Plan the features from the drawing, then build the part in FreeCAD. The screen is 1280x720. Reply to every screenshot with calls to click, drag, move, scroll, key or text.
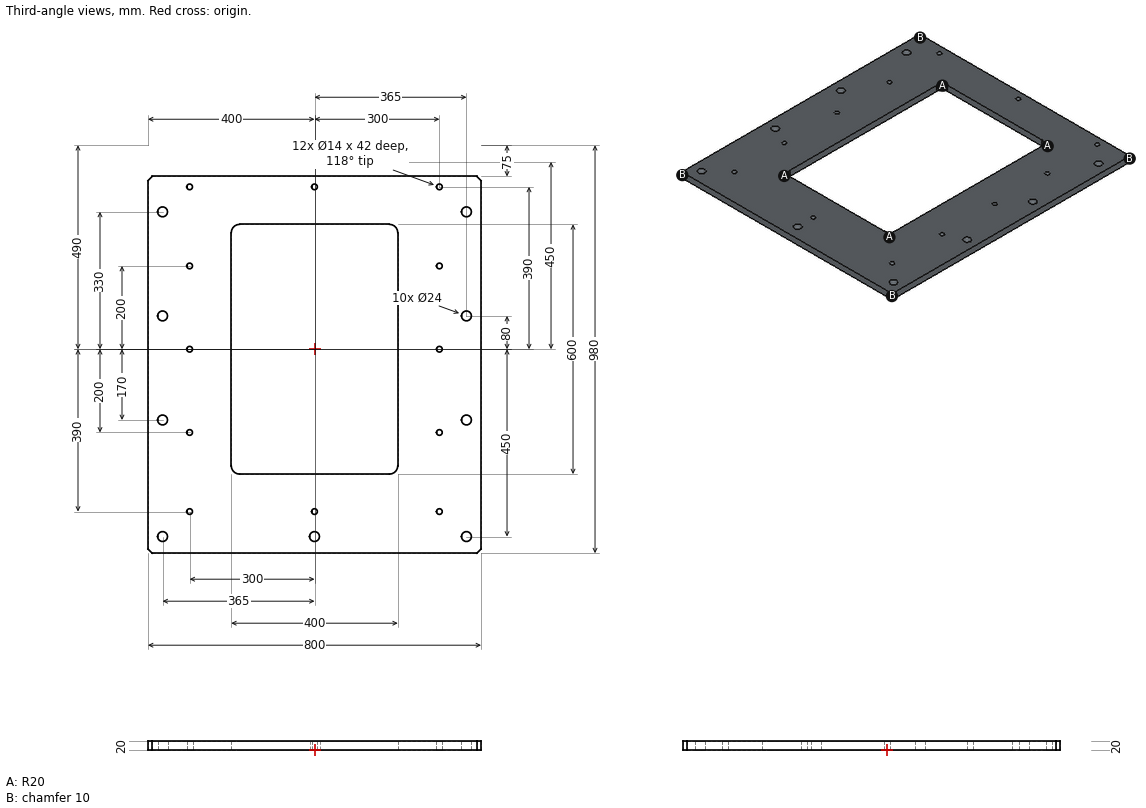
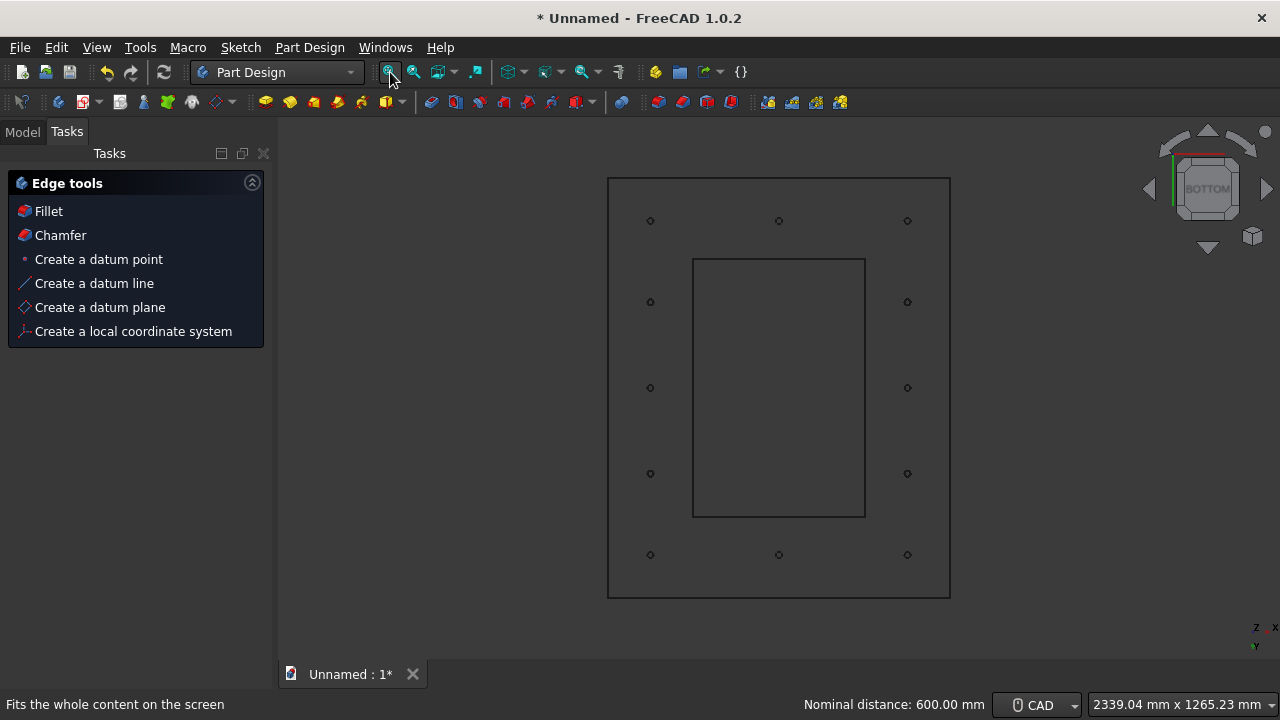
scroll(693, 258, up, 8)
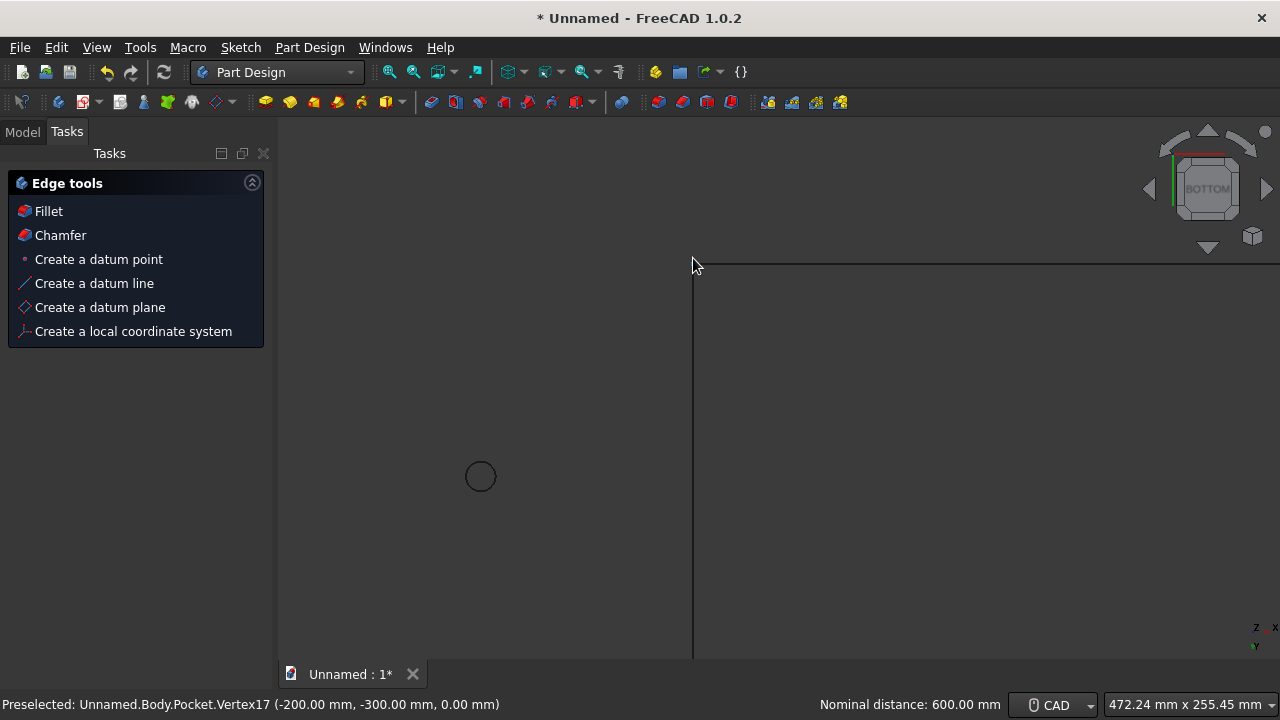
click(390, 72)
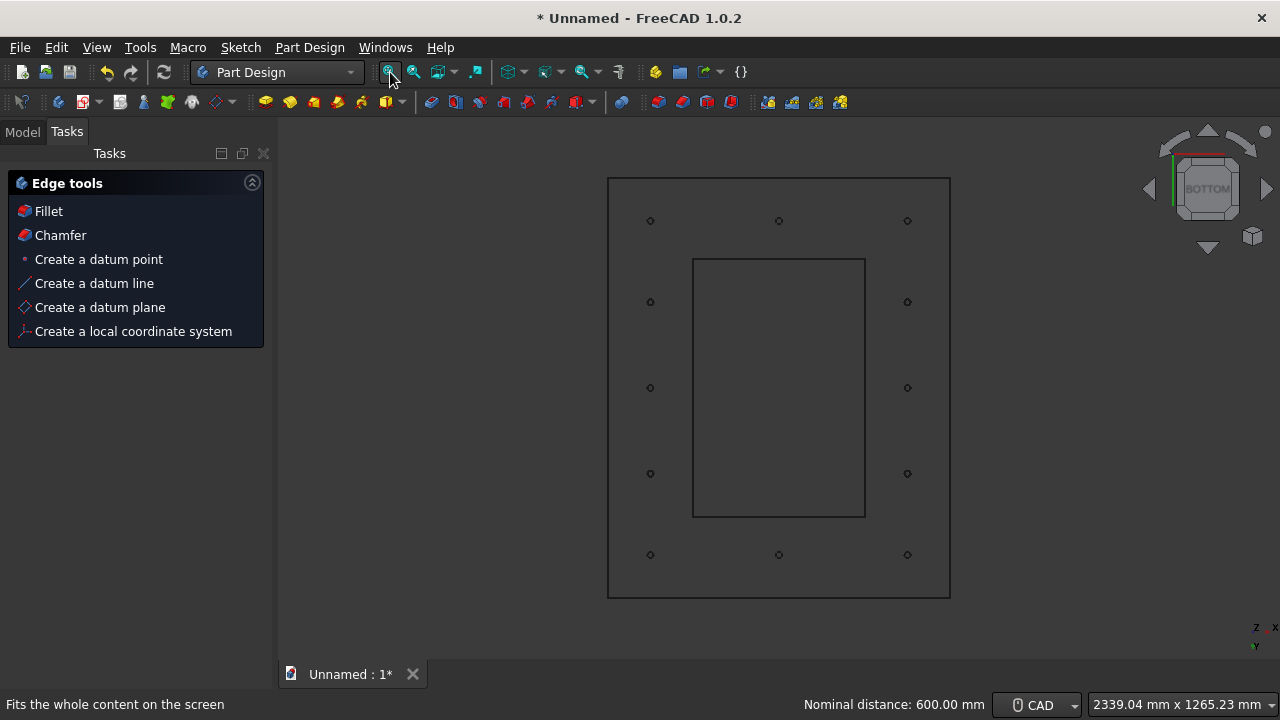
key(4)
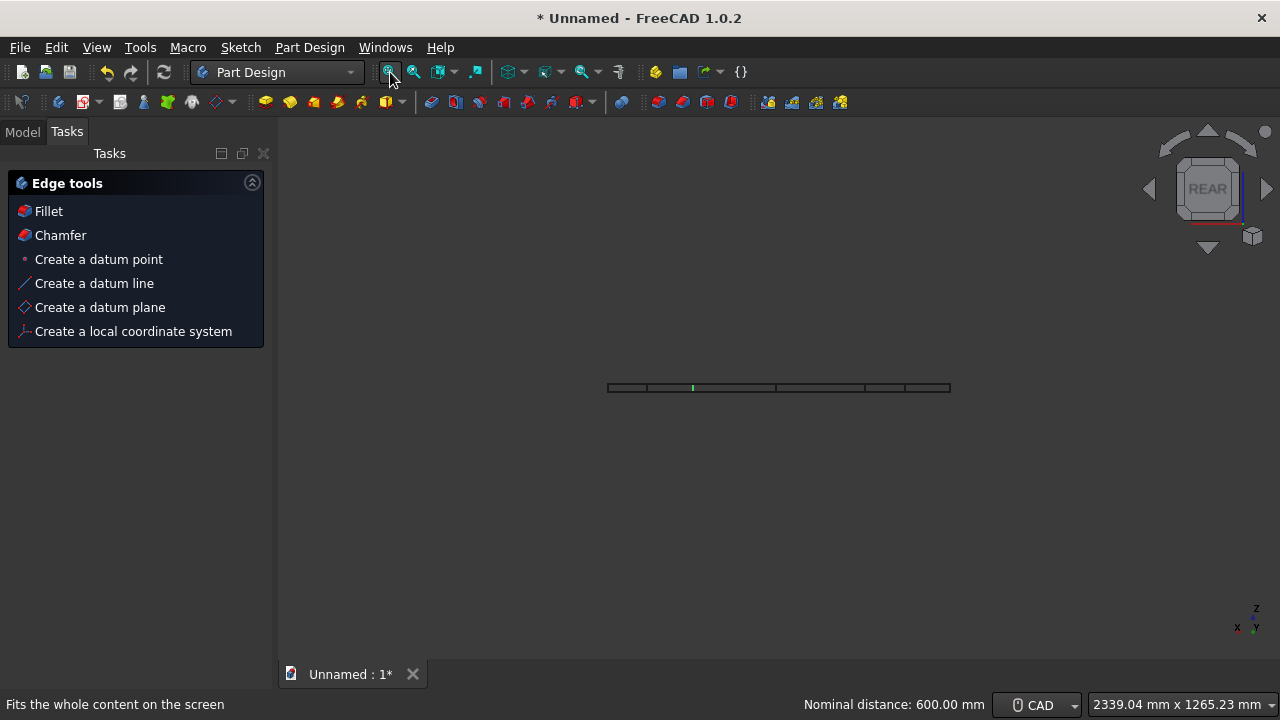
click(390, 72)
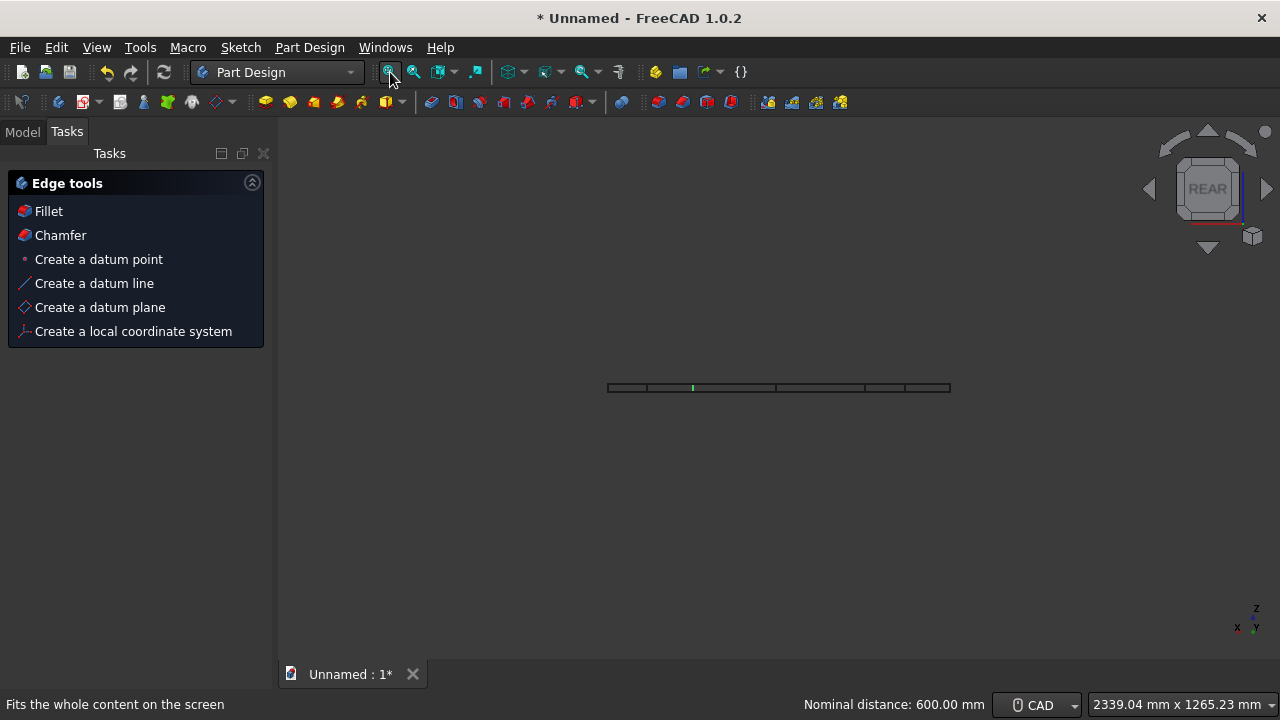
scroll(865, 387, up, 8)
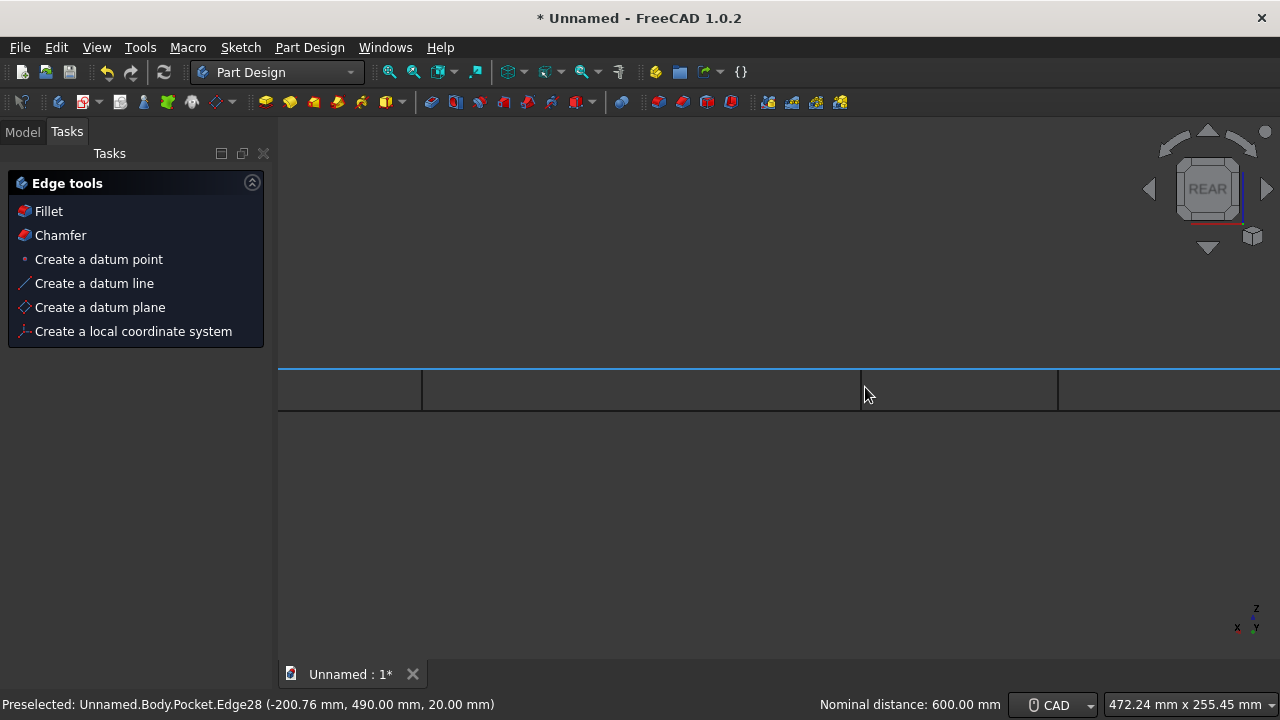
click(861, 389, ctrl)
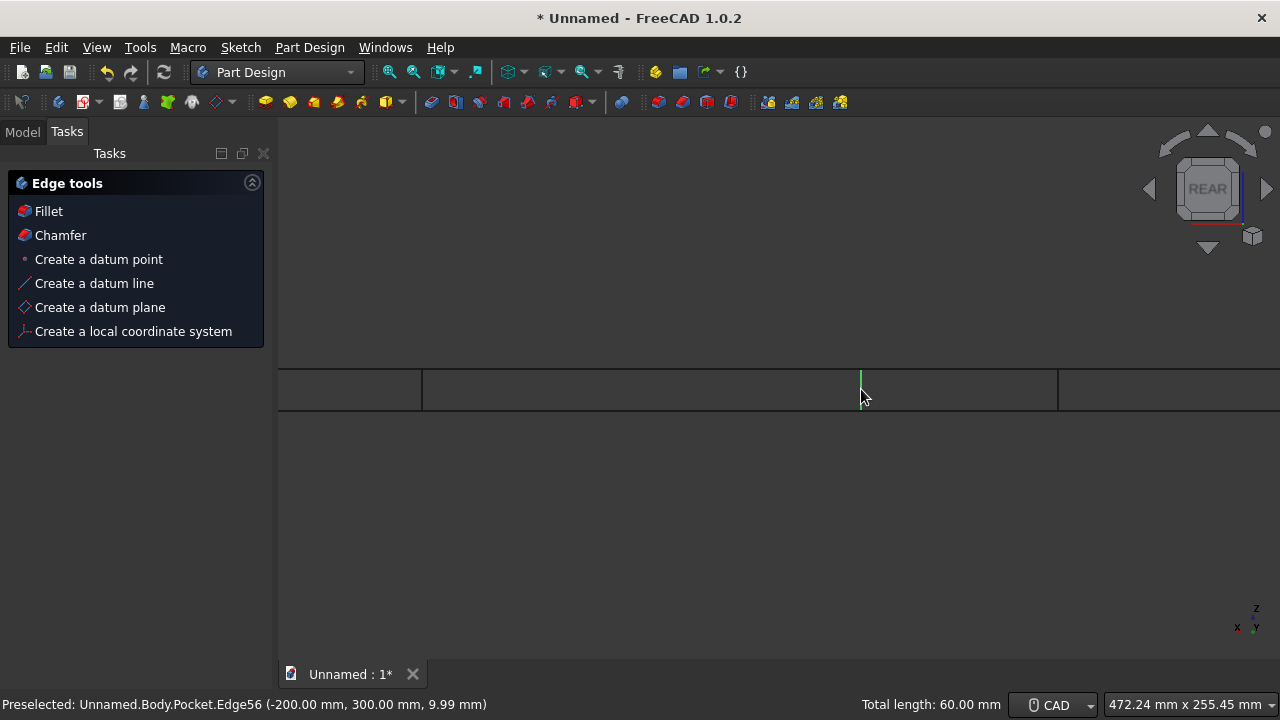
click(390, 72)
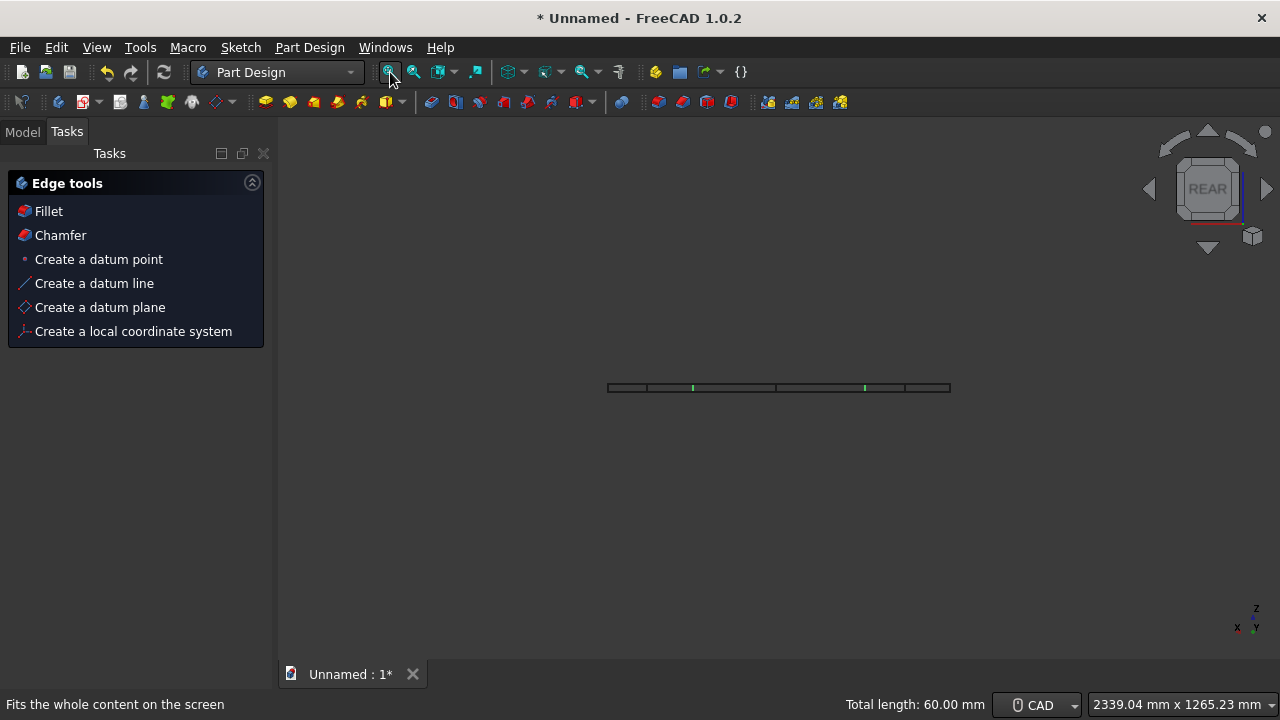
key(6)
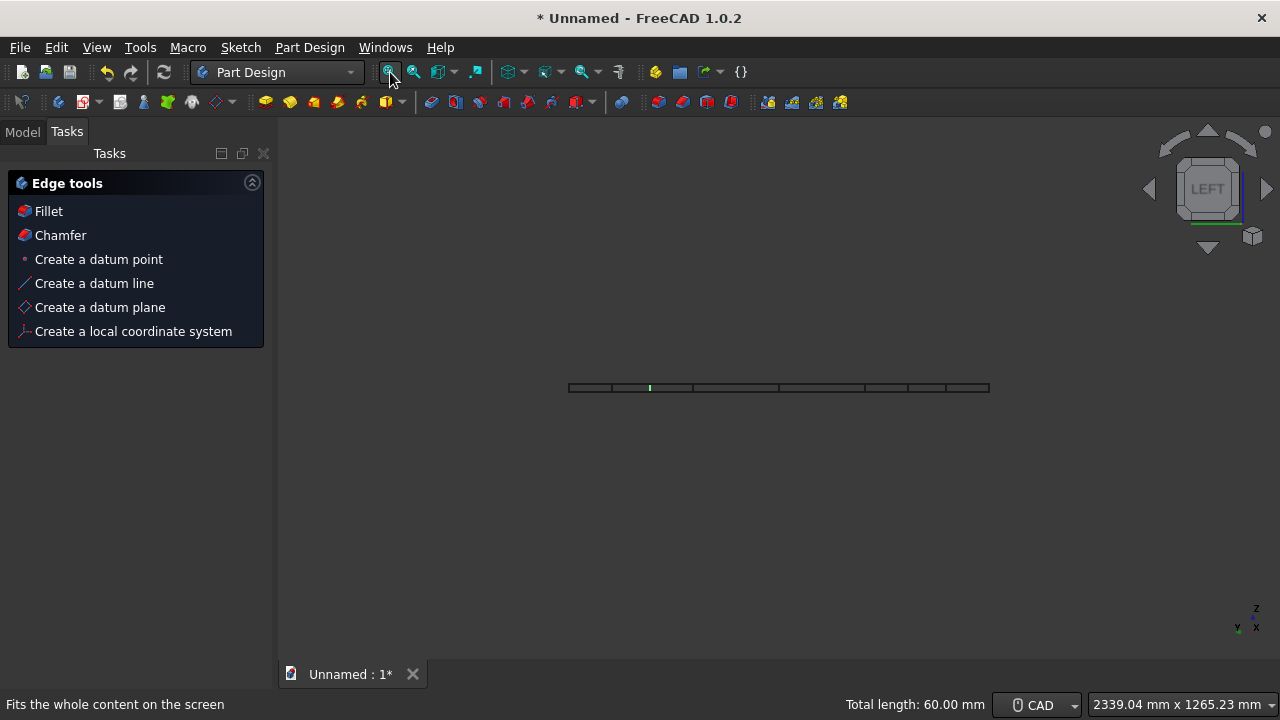
click(390, 72)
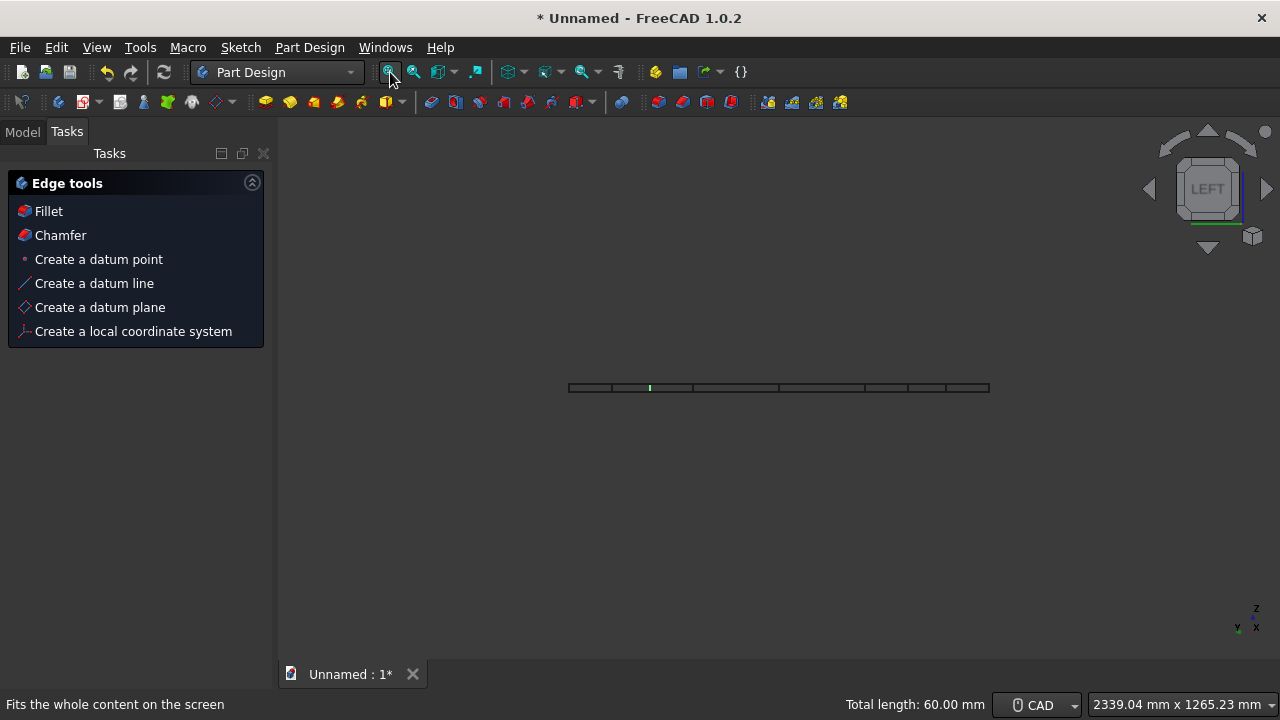
scroll(908, 387, up, 8)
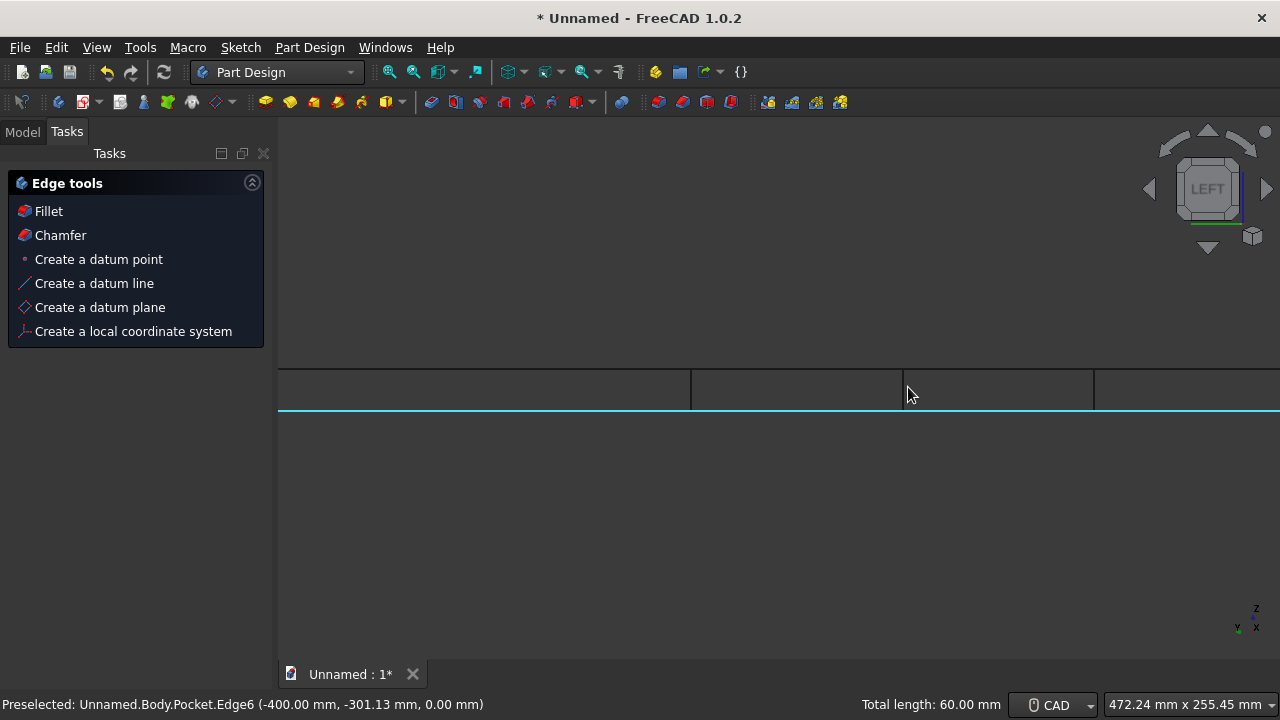
click(903, 389, ctrl)